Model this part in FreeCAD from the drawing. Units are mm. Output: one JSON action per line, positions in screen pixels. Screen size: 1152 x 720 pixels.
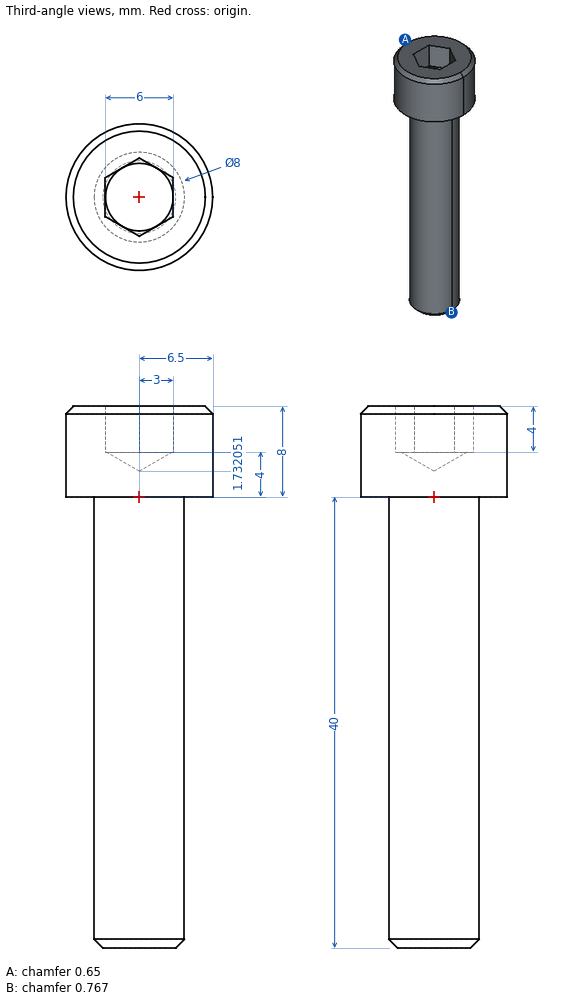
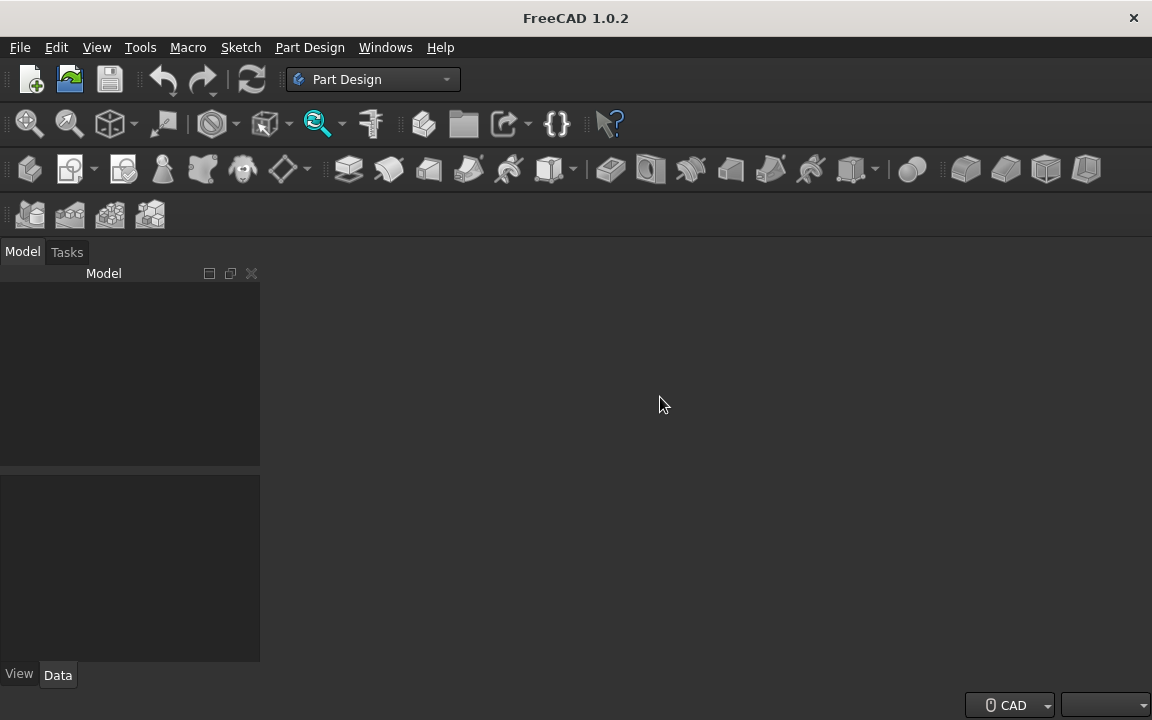
{"action": "left_click", "coordinate": [30, 80]}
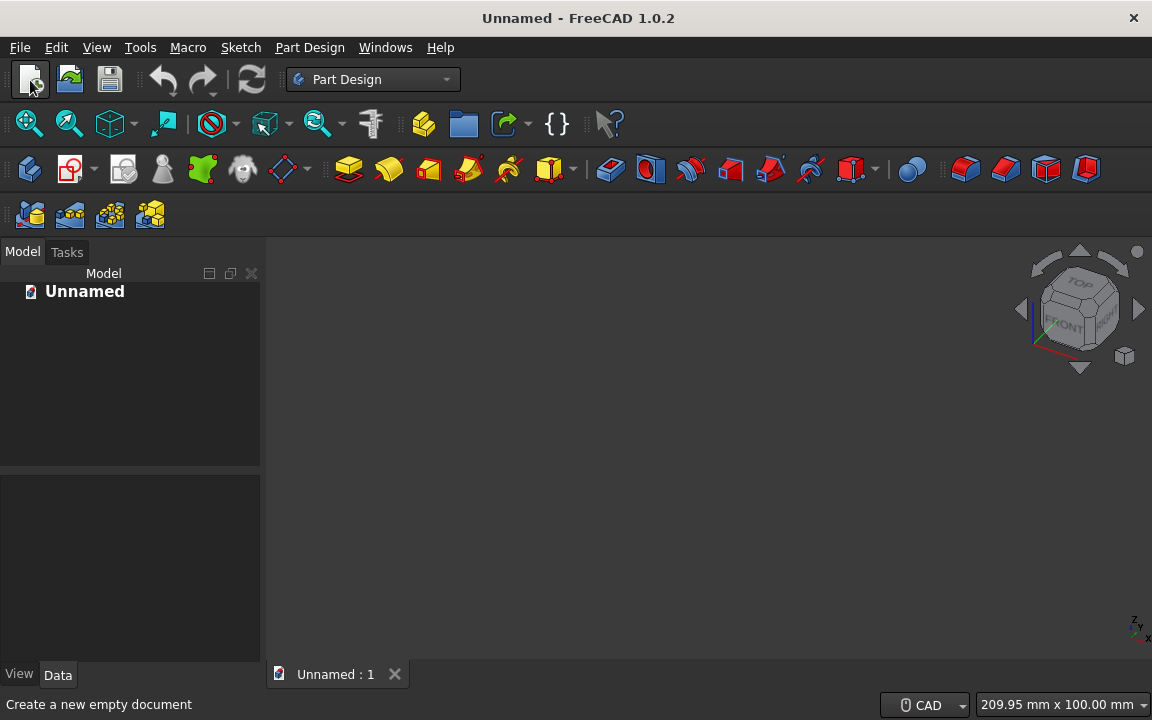
{"action": "left_click", "coordinate": [70, 170]}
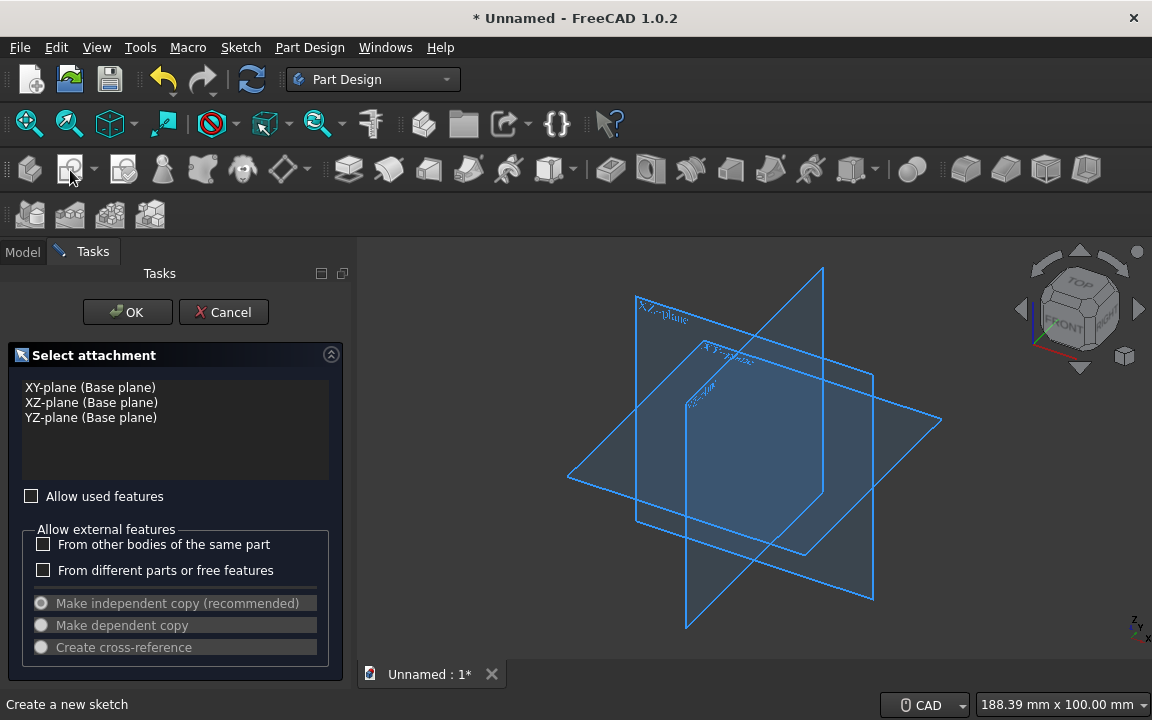
{"action": "left_click", "coordinate": [82, 402]}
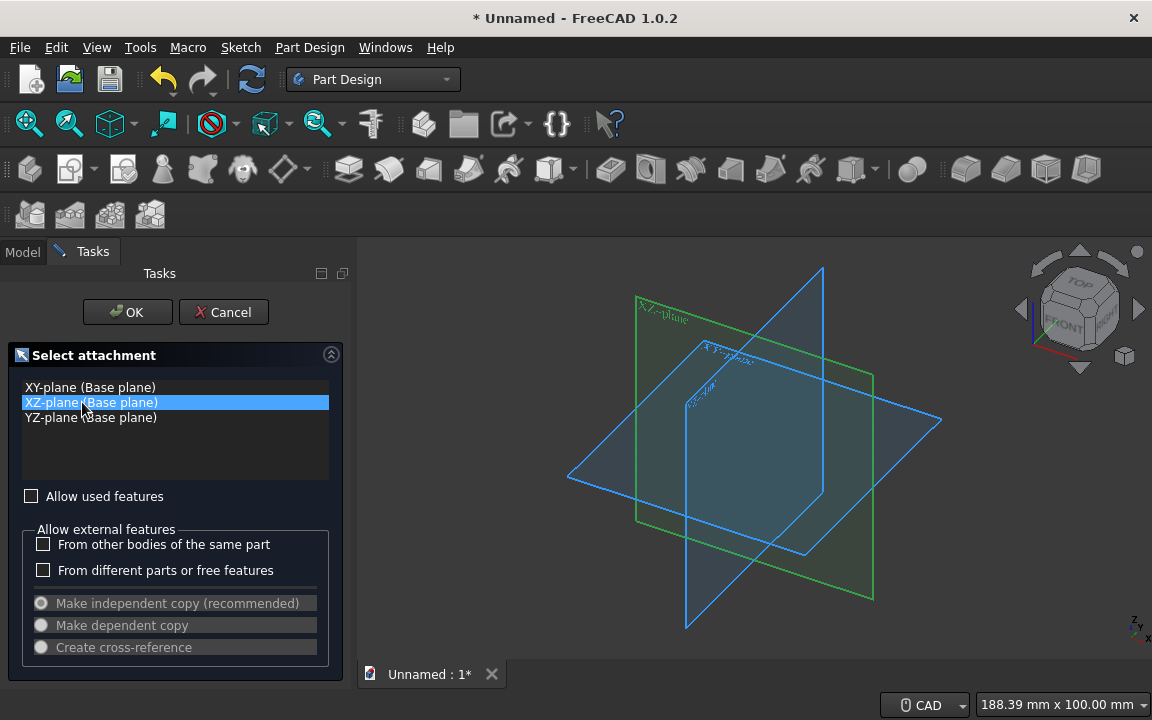
{"action": "left_click", "coordinate": [128, 312]}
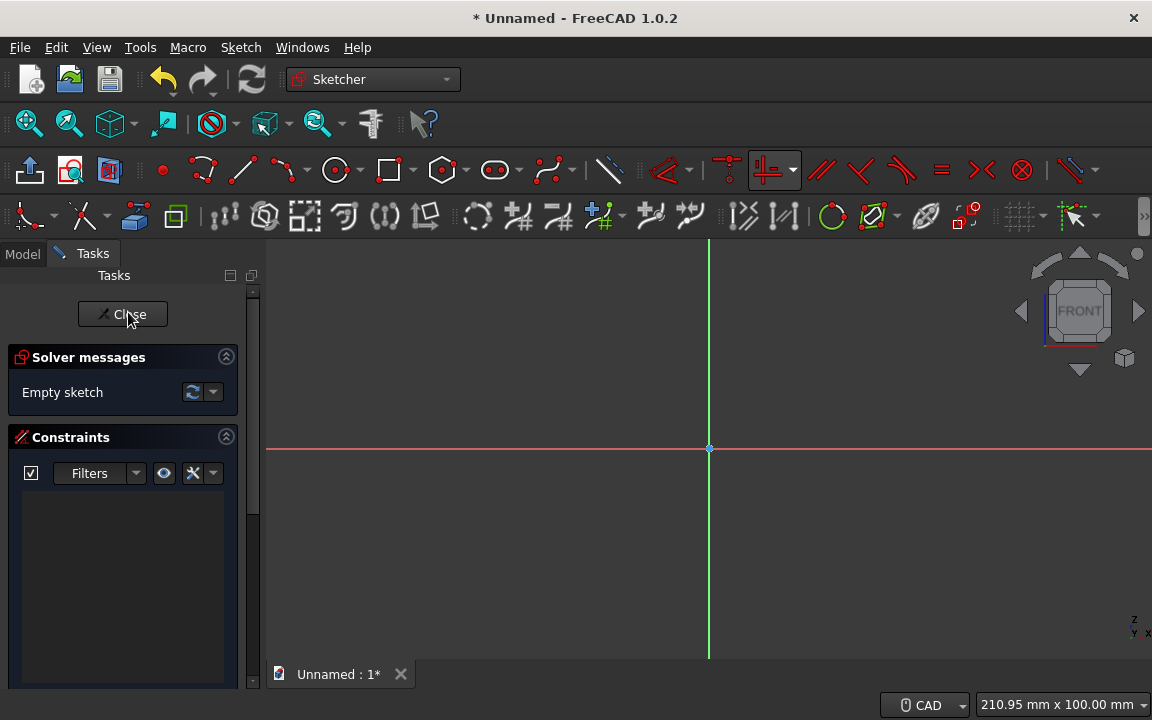
{"action": "scroll", "coordinate": [736, 430], "scroll_direction": "up", "scroll_amount": 10}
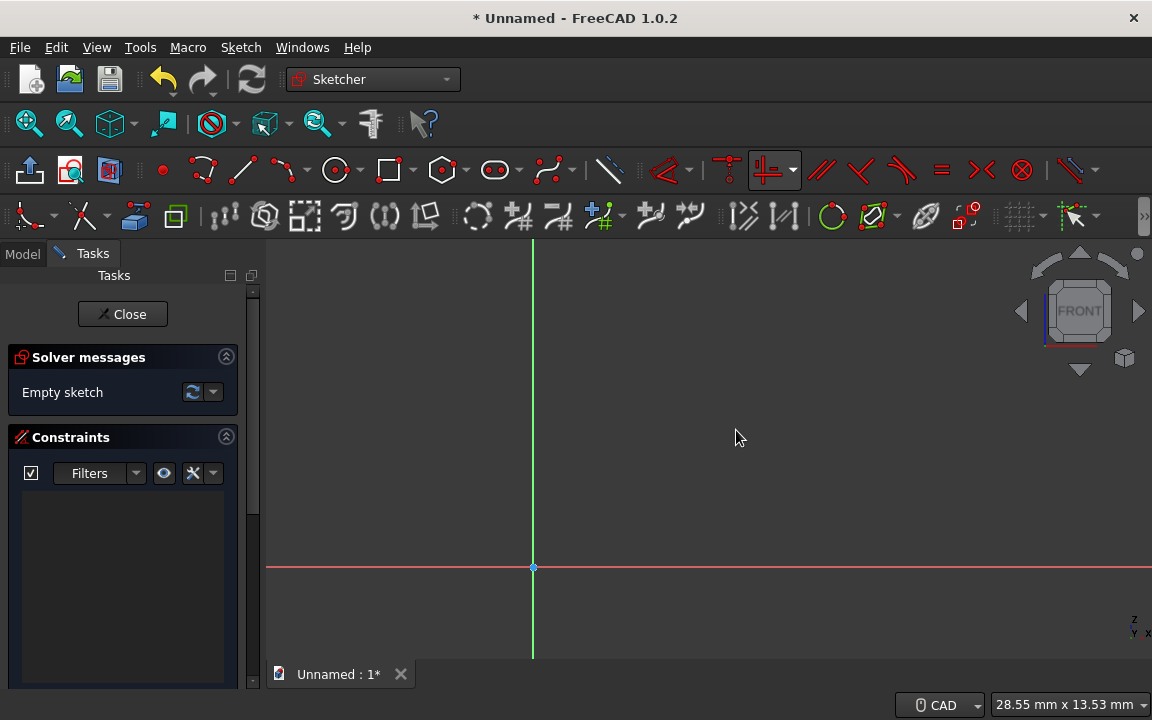
{"action": "left_click", "coordinate": [390, 170]}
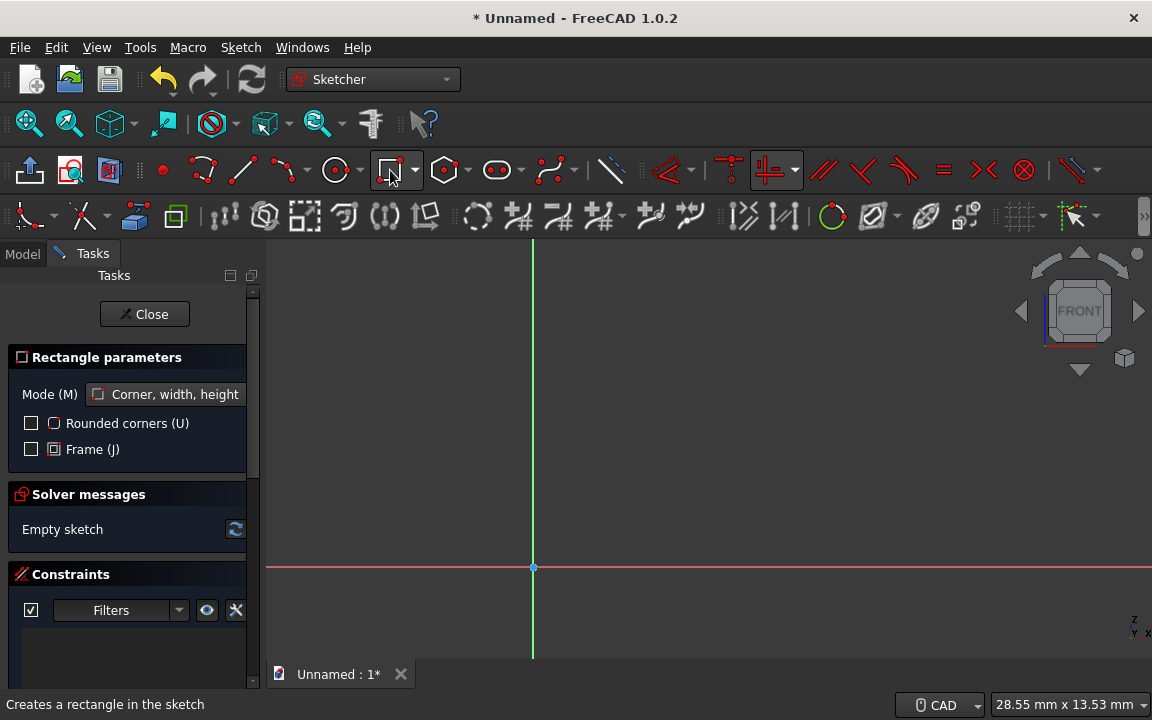
{"action": "left_click", "coordinate": [533, 567]}
{"action": "mouse_move", "coordinate": [735, 319]}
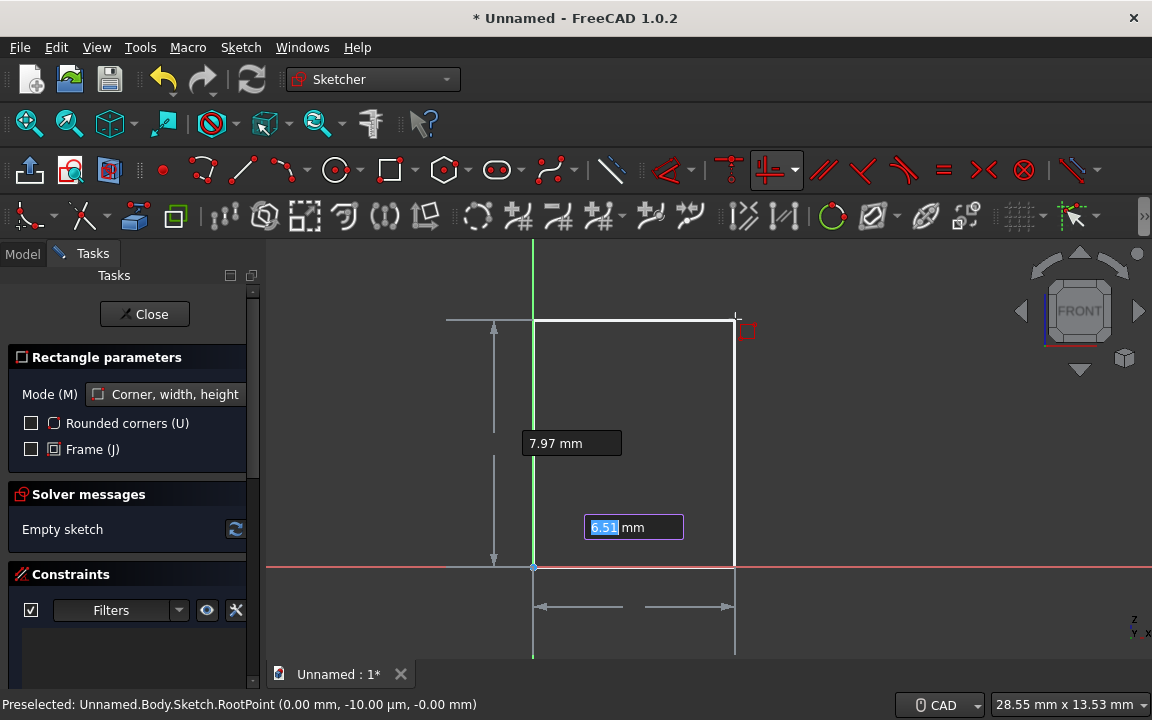
{"action": "type", "text": "6.5"}
{"action": "key", "text": "Tab"}
{"action": "type", "text": "8"}
{"action": "key", "text": "Return"}
{"action": "key", "text": "Escape"}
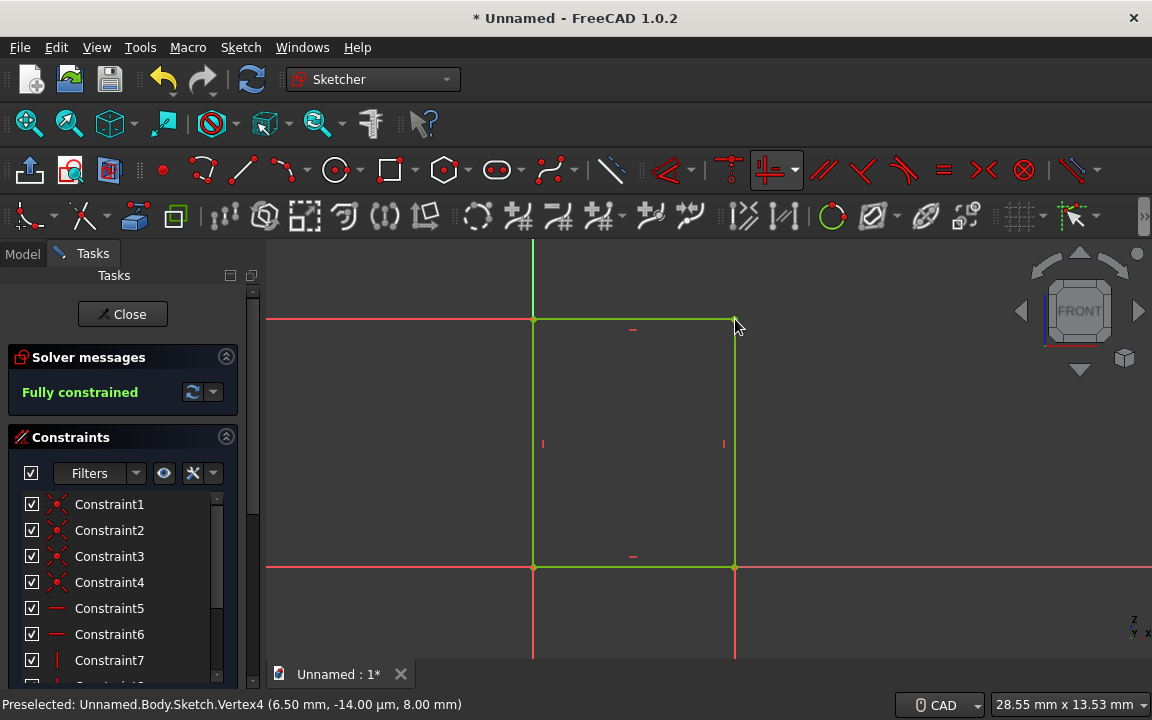
{"action": "left_click", "coordinate": [123, 314]}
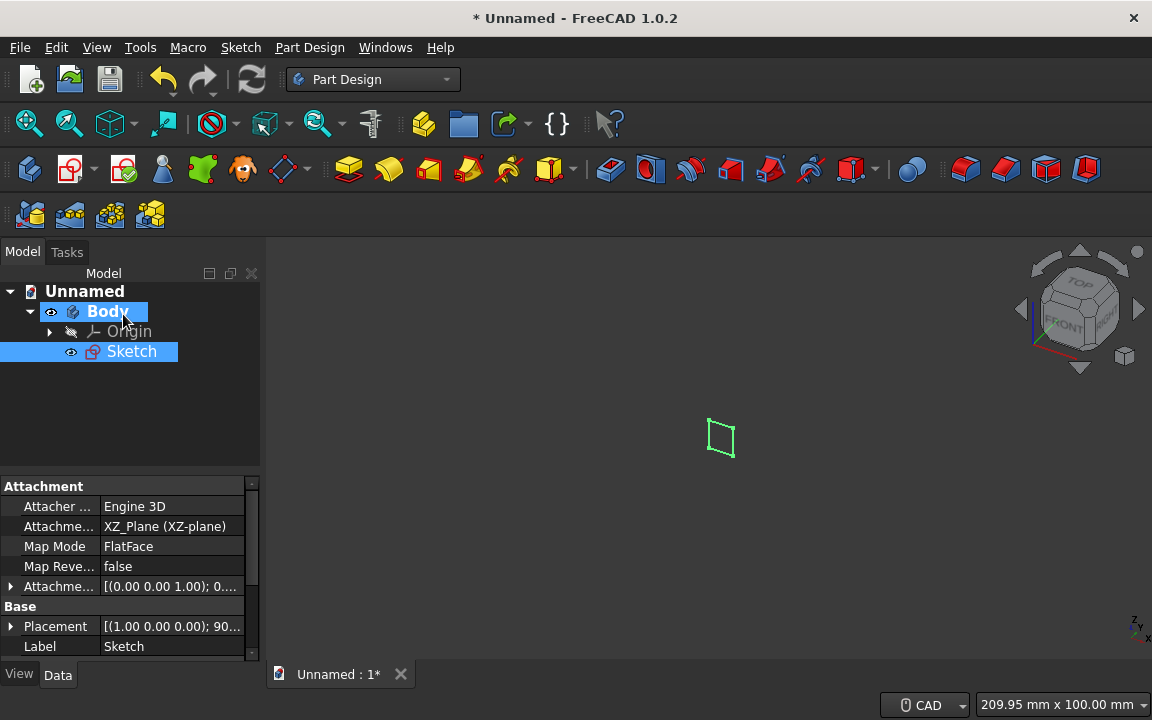
{"action": "left_click", "coordinate": [390, 170]}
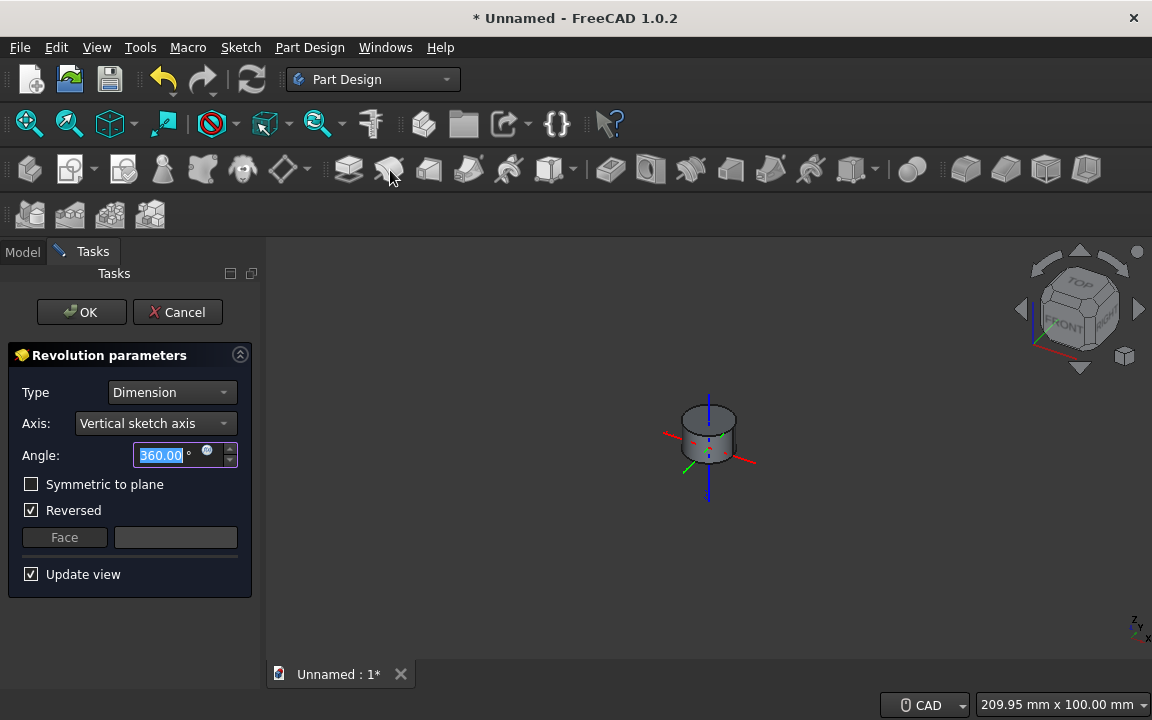
{"action": "left_click", "coordinate": [82, 312]}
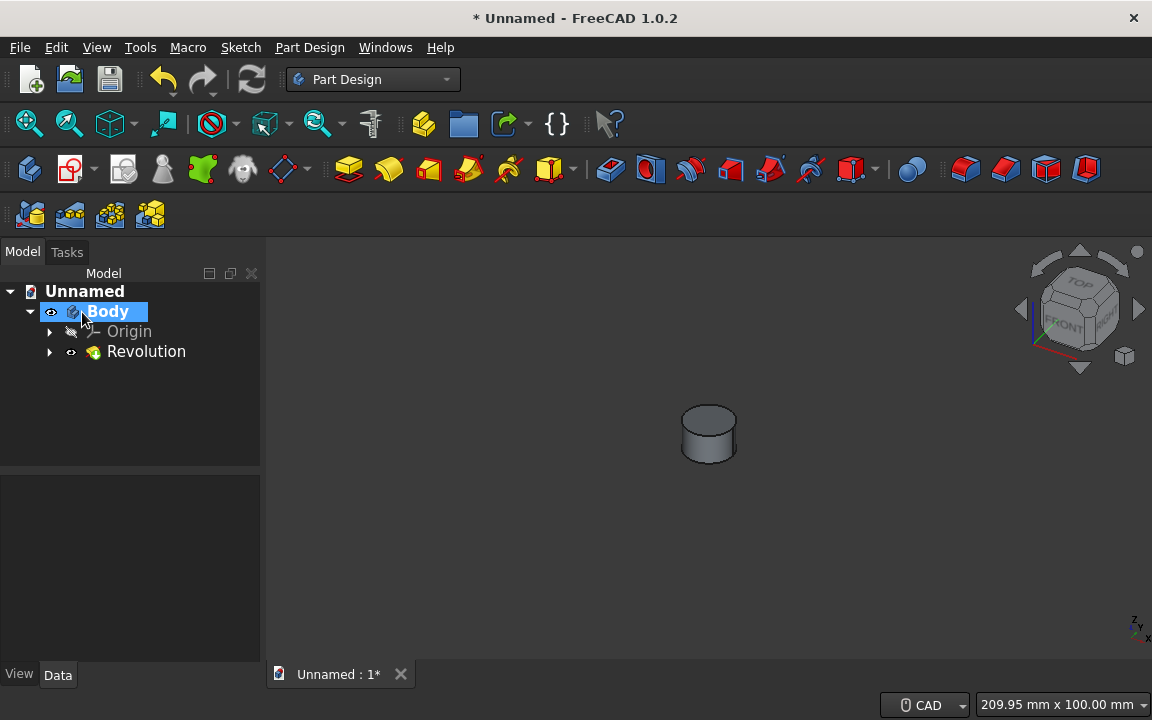
{"action": "left_click", "coordinate": [30, 124]}